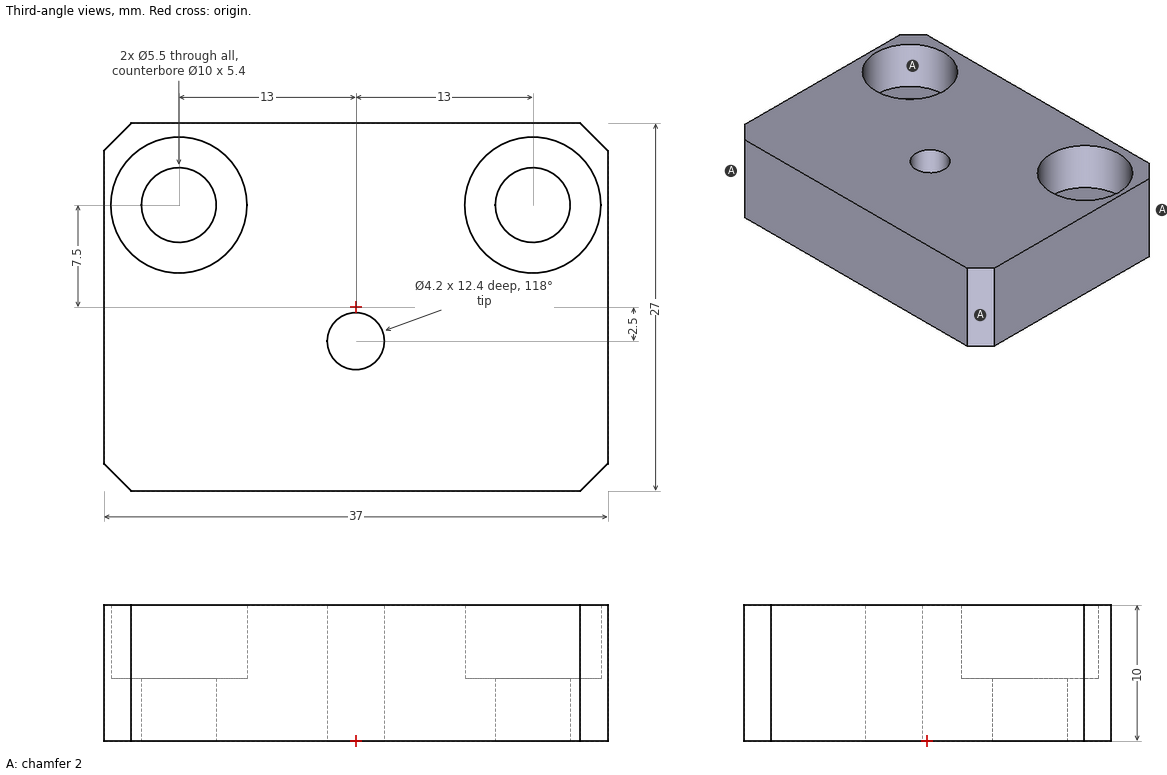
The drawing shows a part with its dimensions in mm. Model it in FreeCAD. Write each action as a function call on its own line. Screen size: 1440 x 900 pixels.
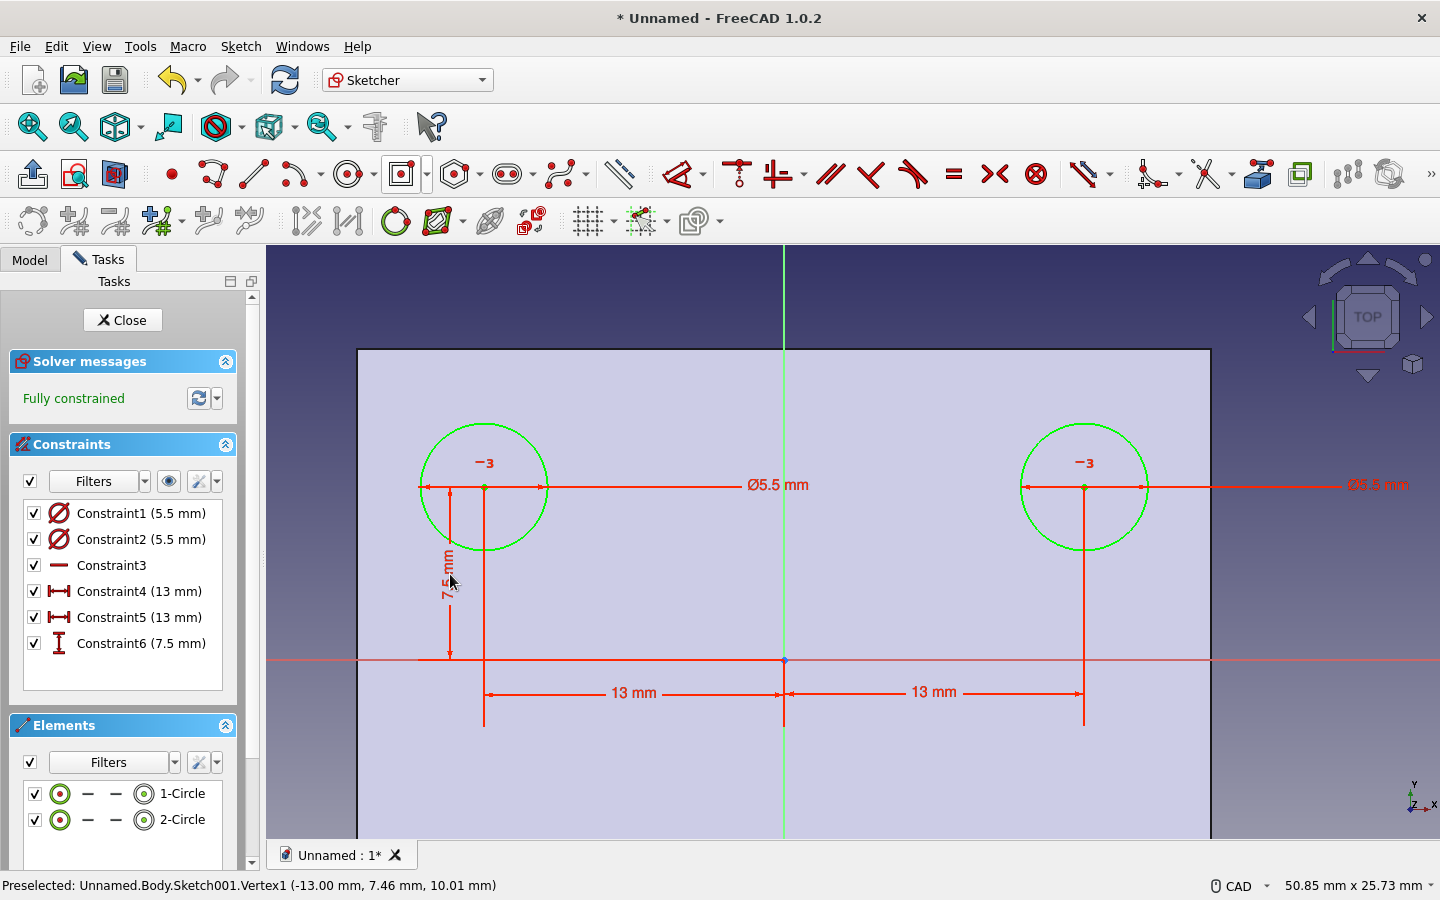
click(123, 320)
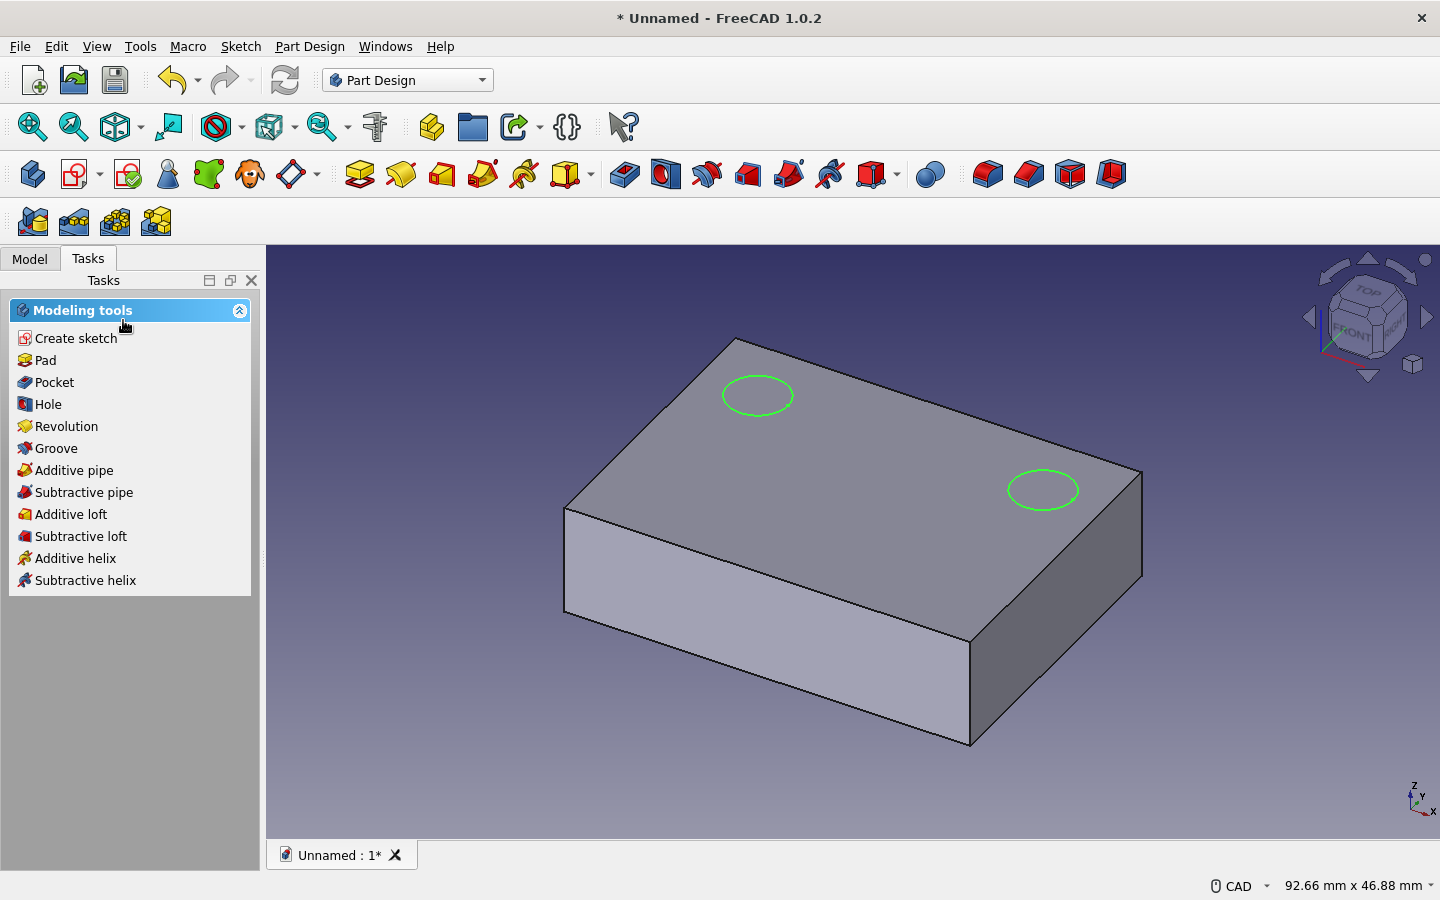
click(666, 174)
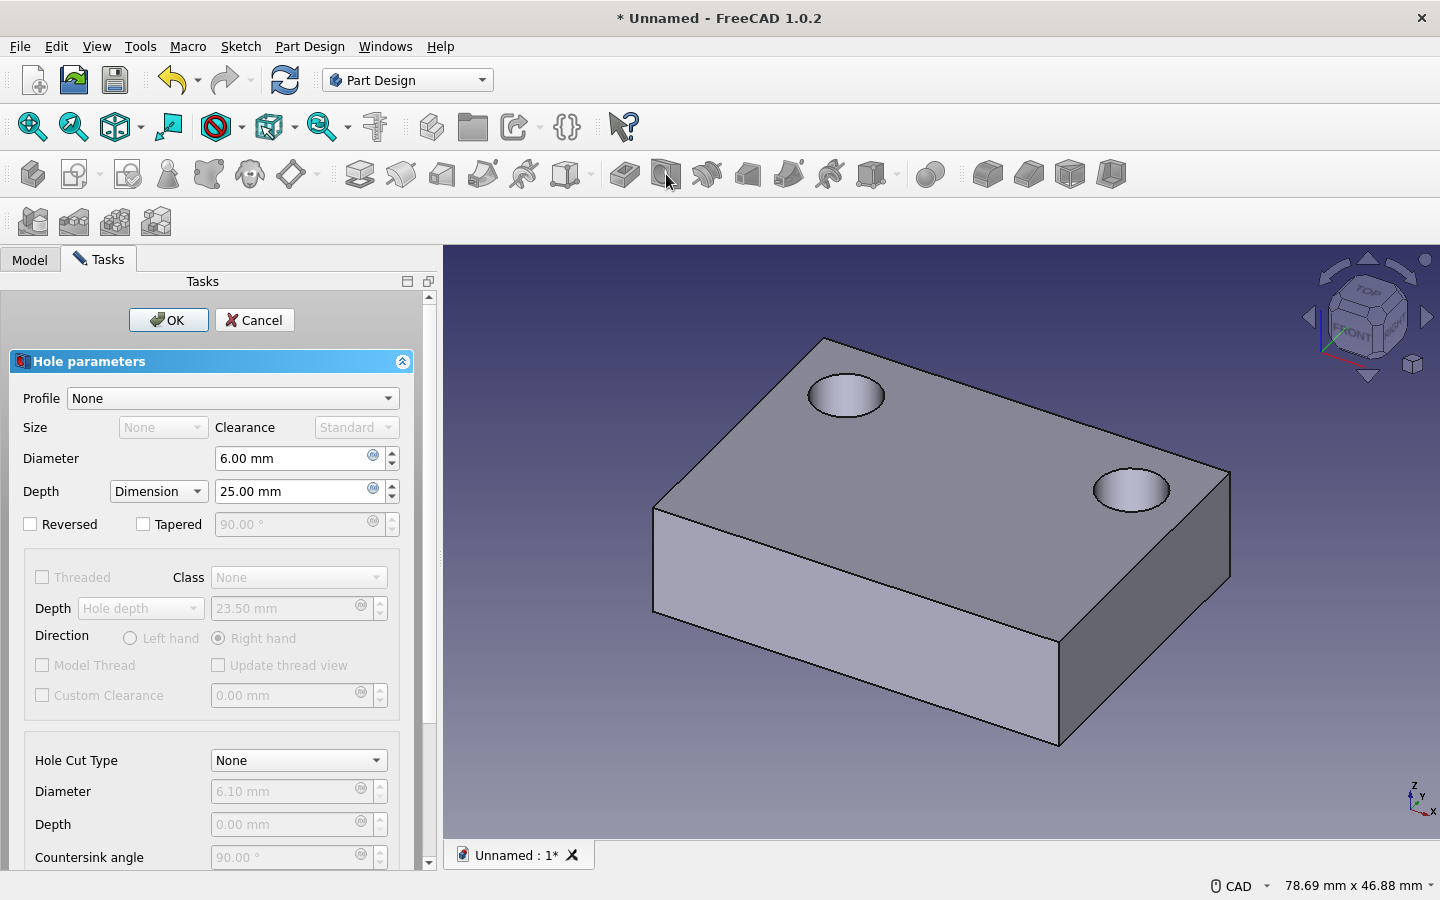
triple_click(300, 458)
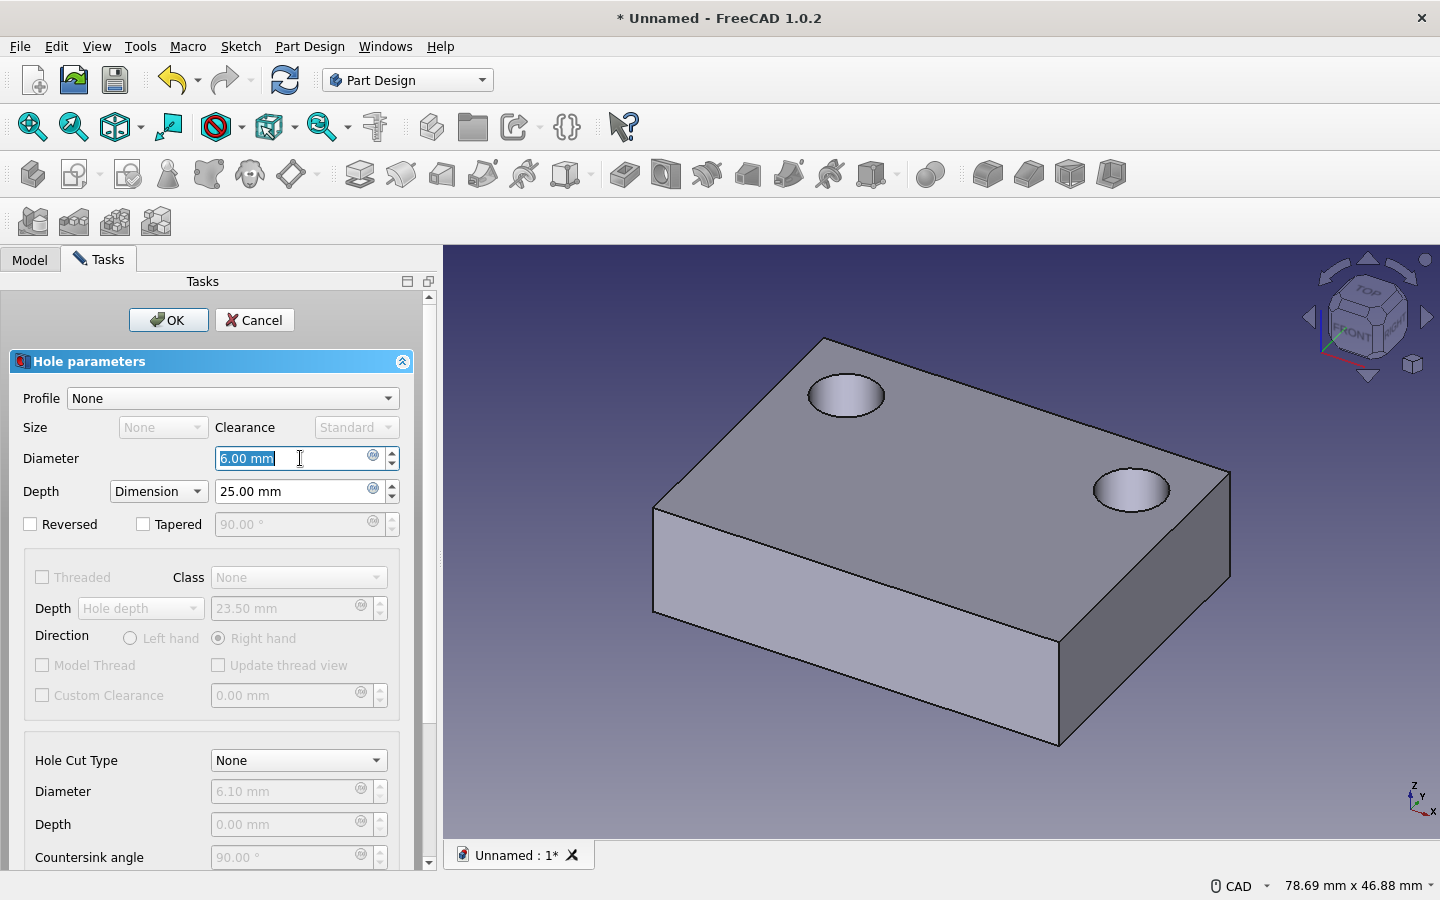
text(5.5)
key(Tab)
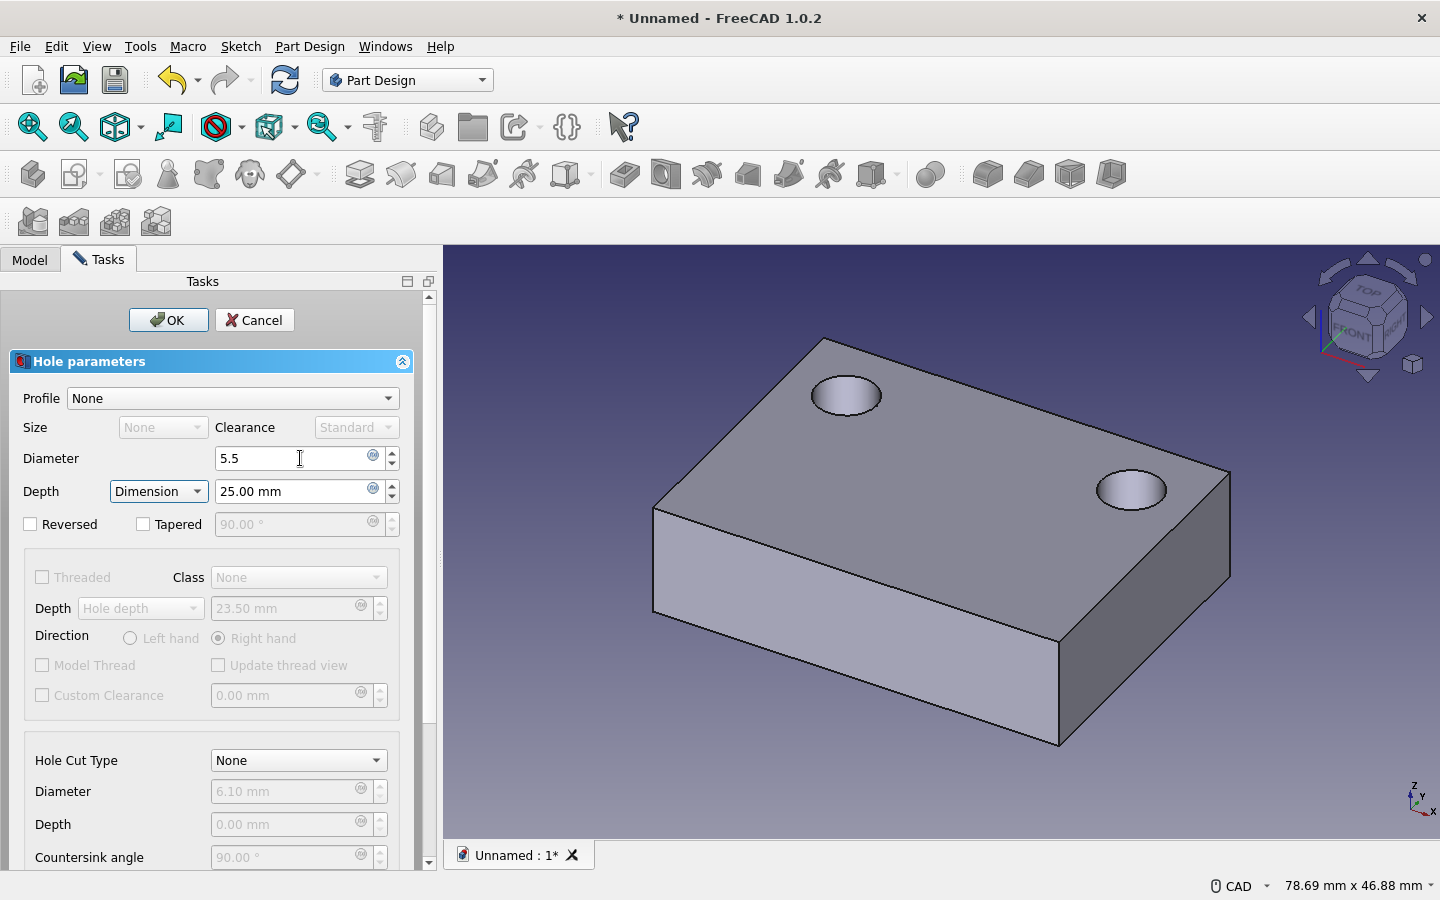
click(160, 492)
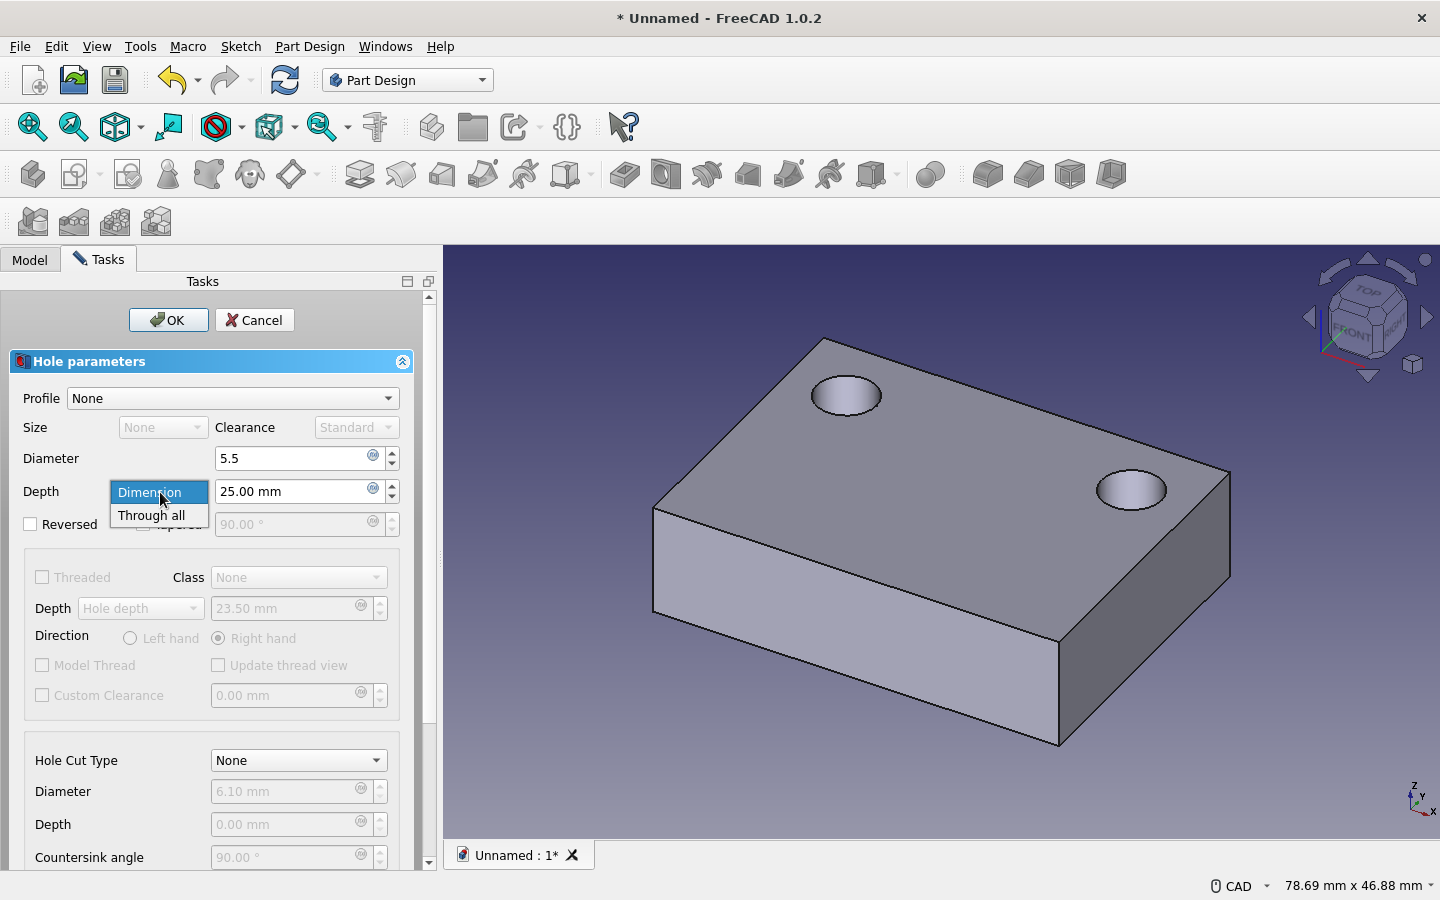
click(158, 516)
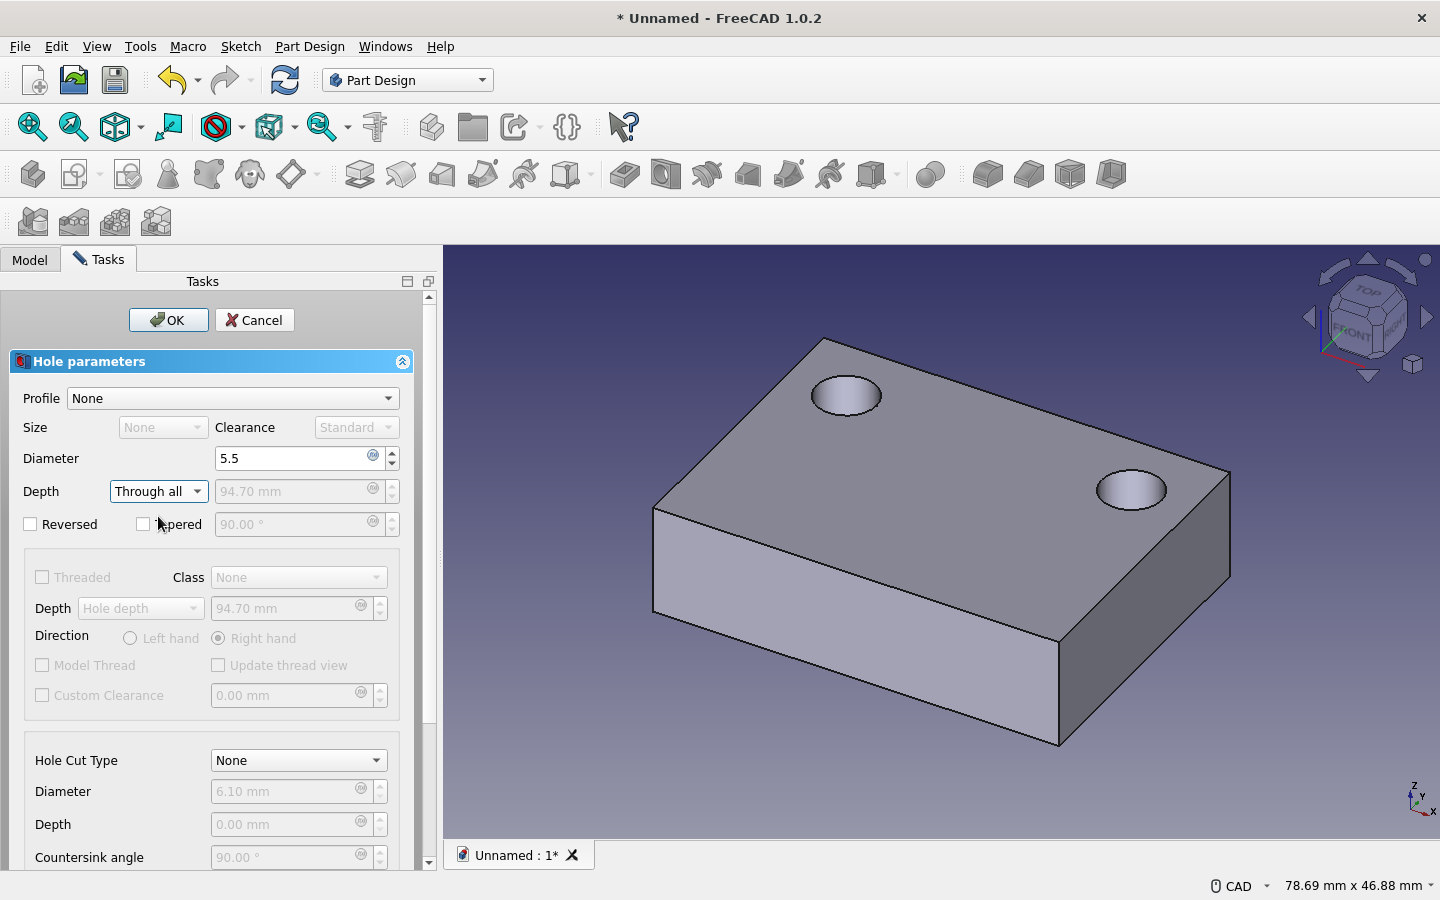
click(300, 760)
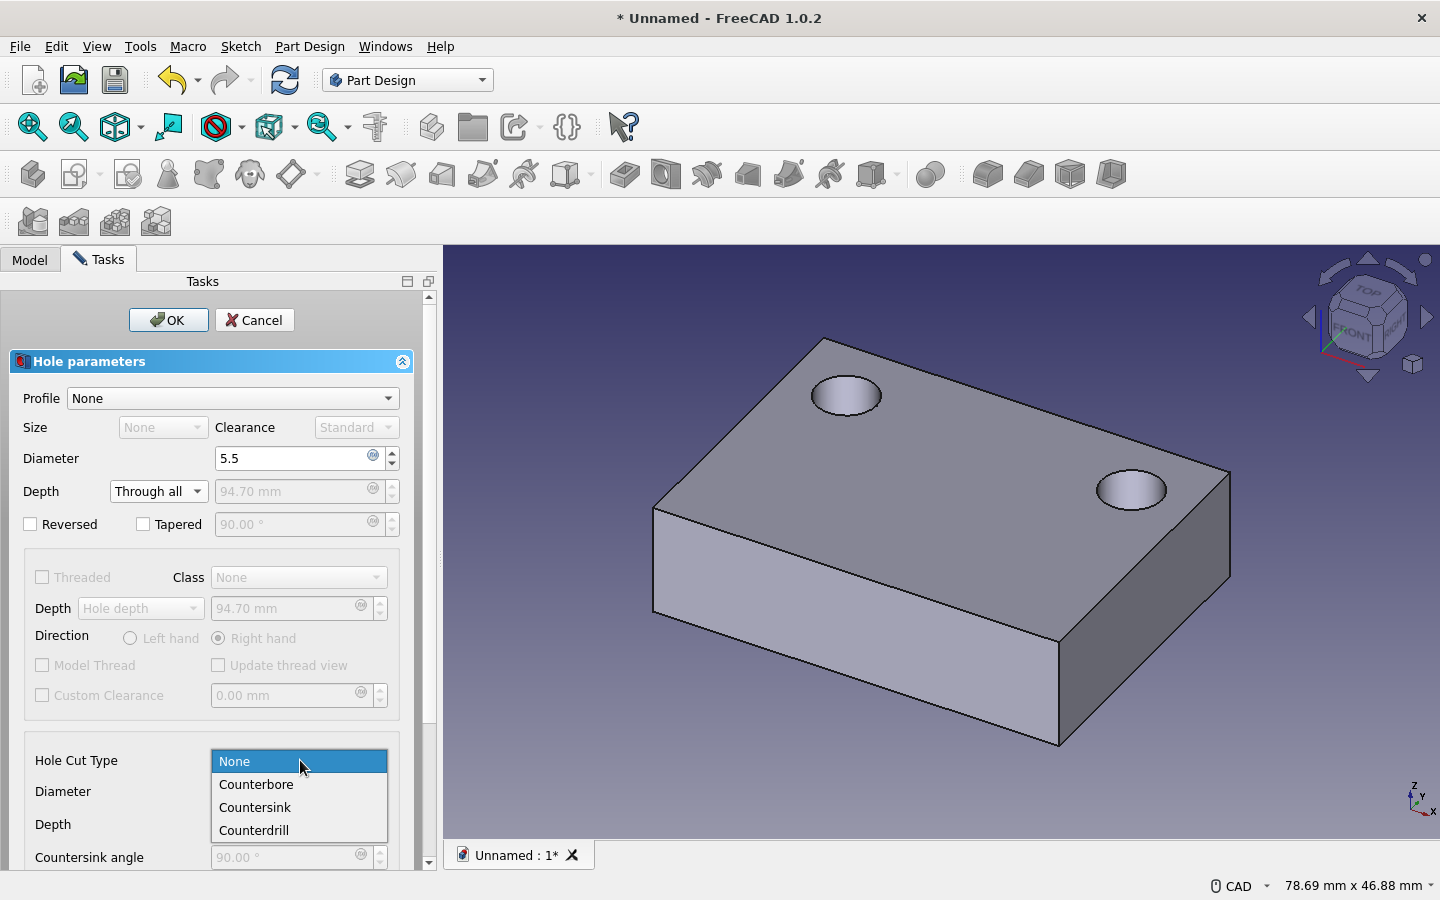
click(298, 784)